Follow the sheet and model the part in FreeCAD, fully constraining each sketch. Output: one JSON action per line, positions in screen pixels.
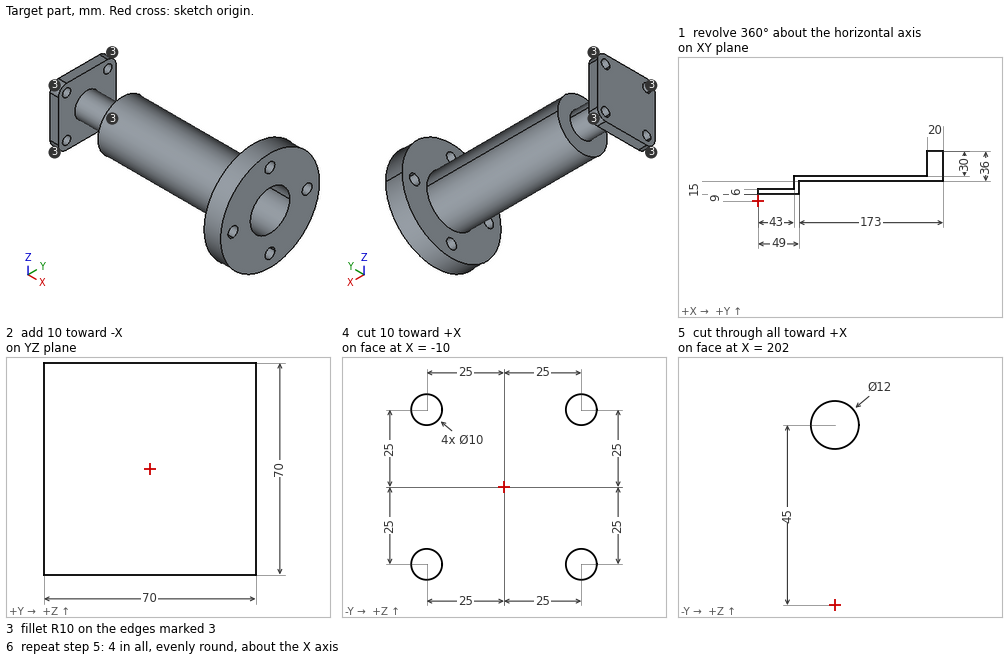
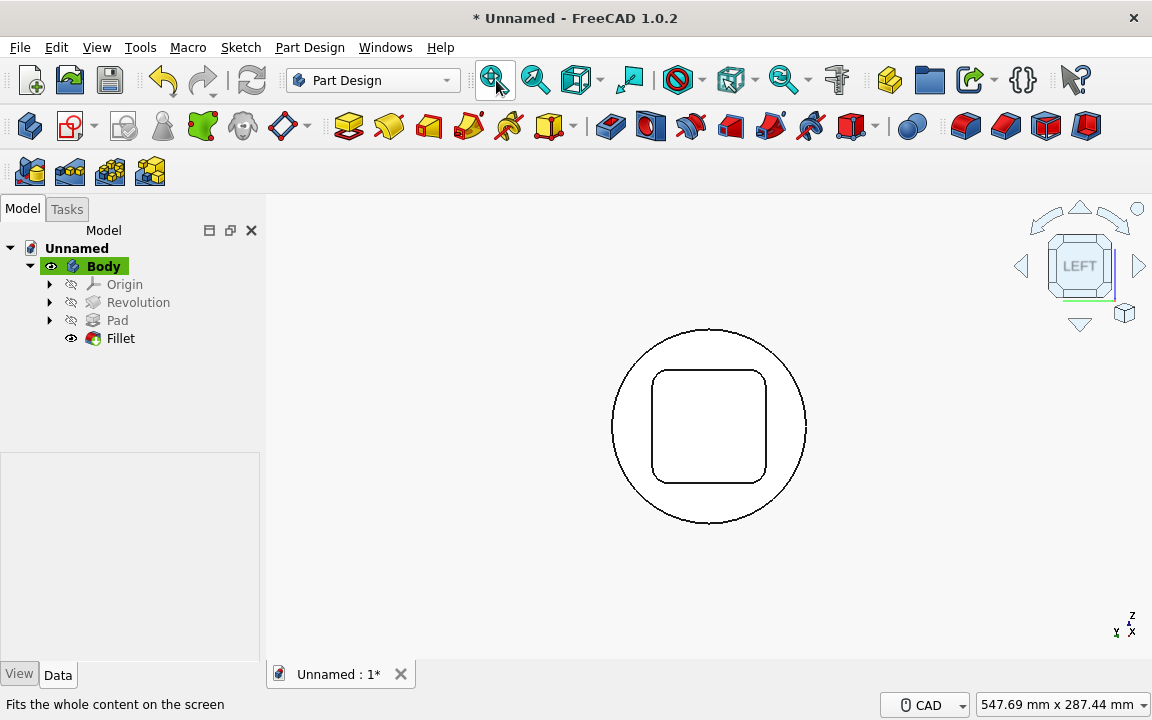
{"action": "left_click", "coordinate": [709, 425]}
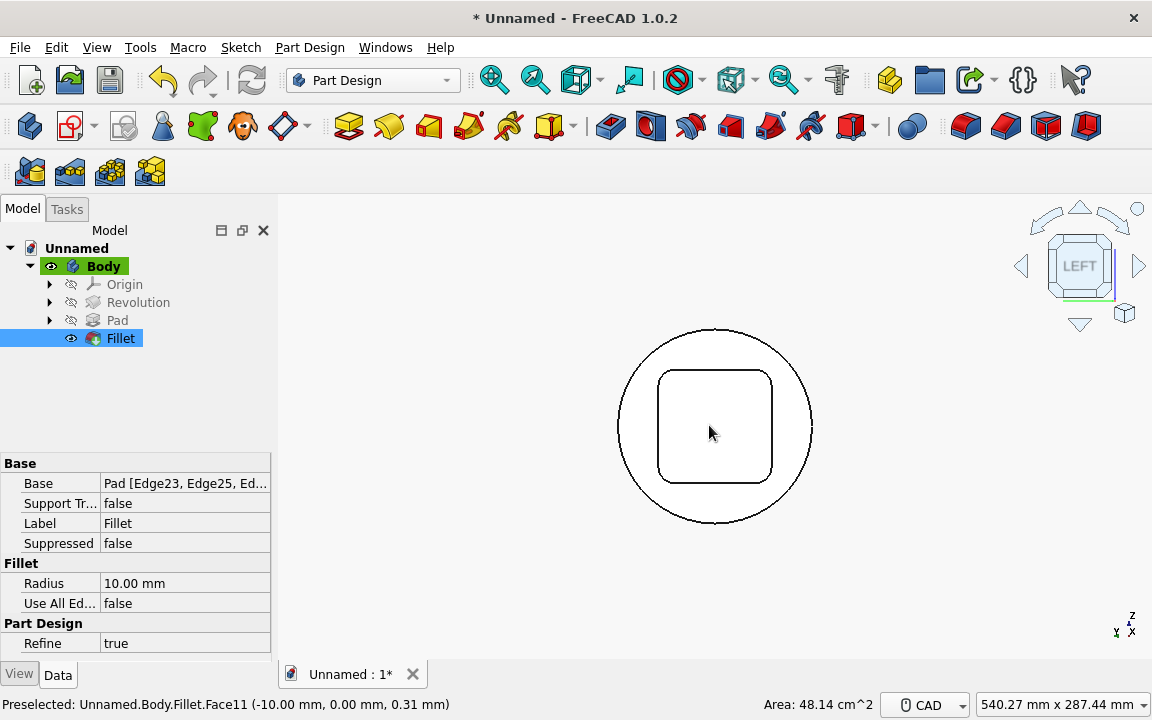
{"action": "left_click", "coordinate": [70, 126]}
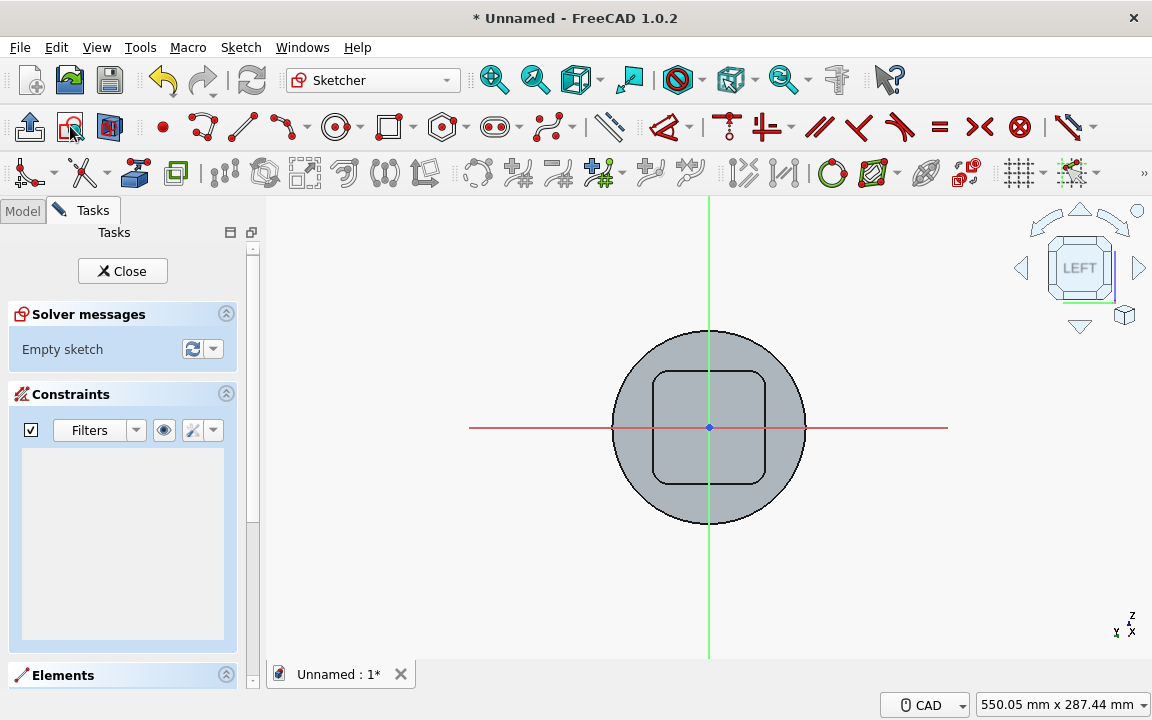
{"action": "scroll", "coordinate": [749, 428], "scroll_direction": "up", "scroll_amount": 5}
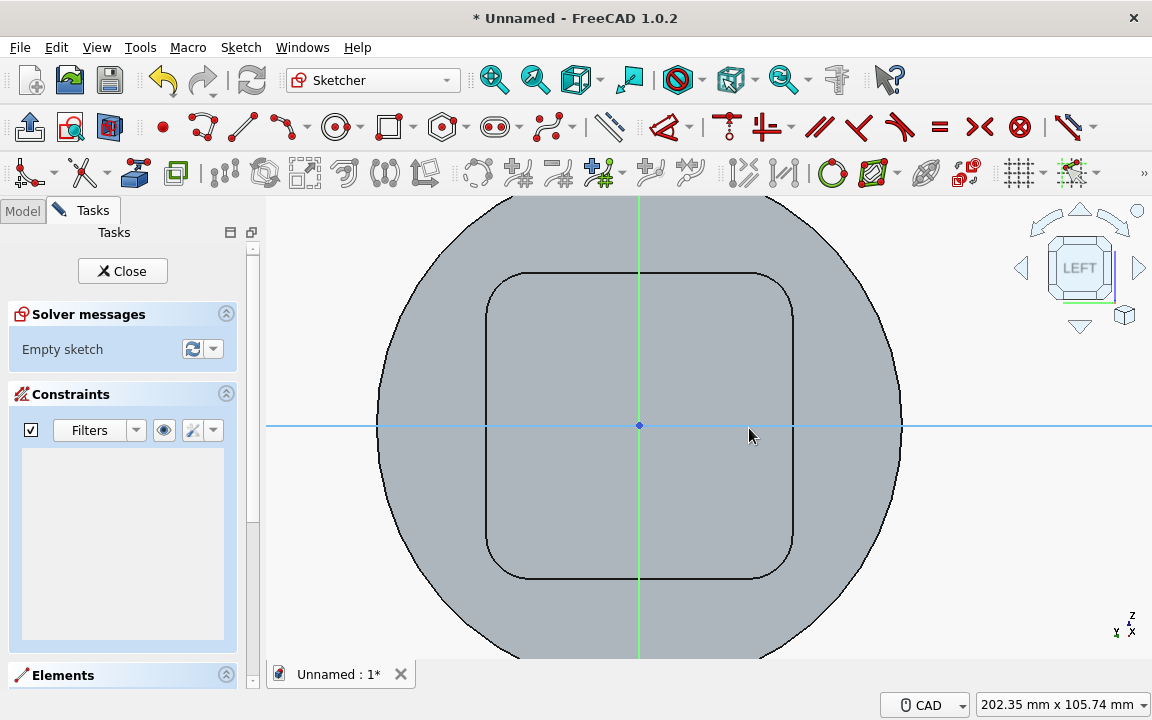
{"action": "key", "text": "g c"}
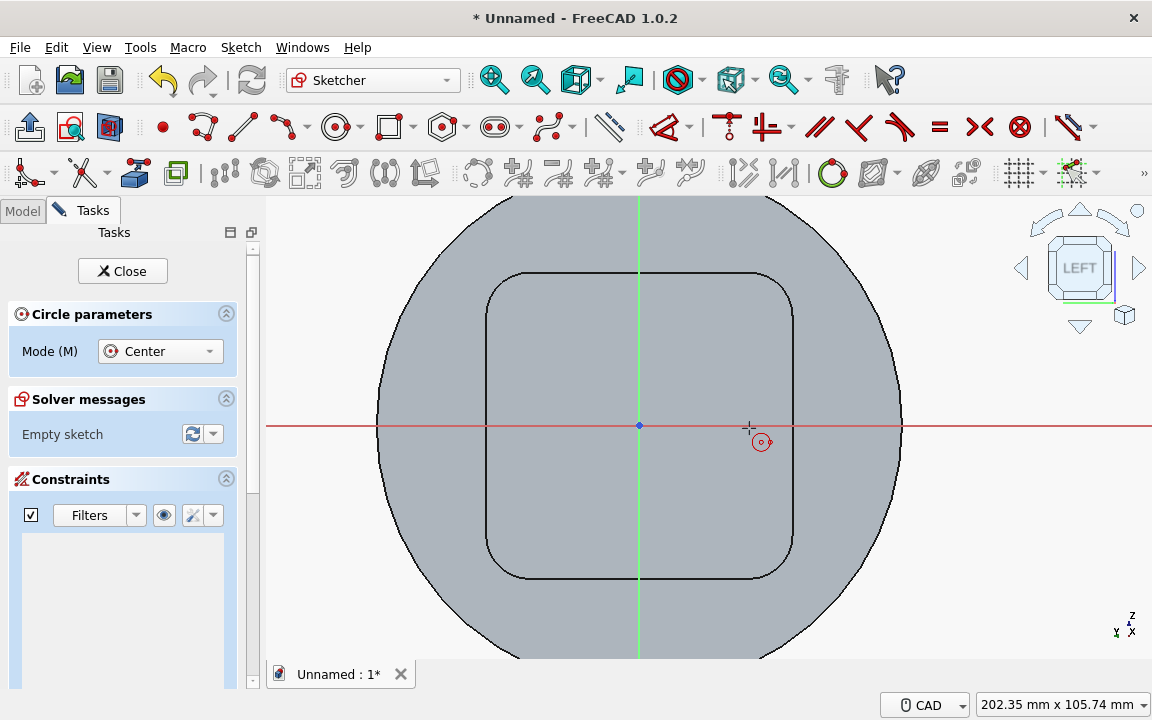
{"action": "left_click", "coordinate": [530, 316]}
{"action": "mouse_move", "coordinate": [545, 301]}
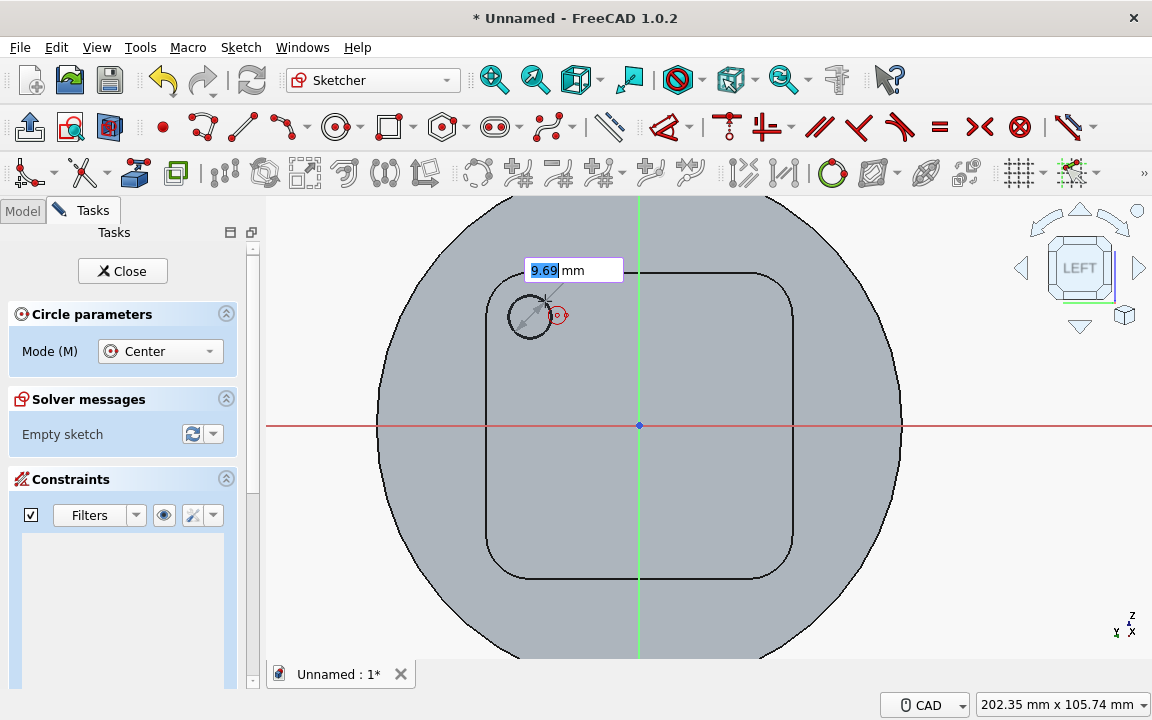
{"action": "type", "text": "10"}
{"action": "key", "text": "Return"}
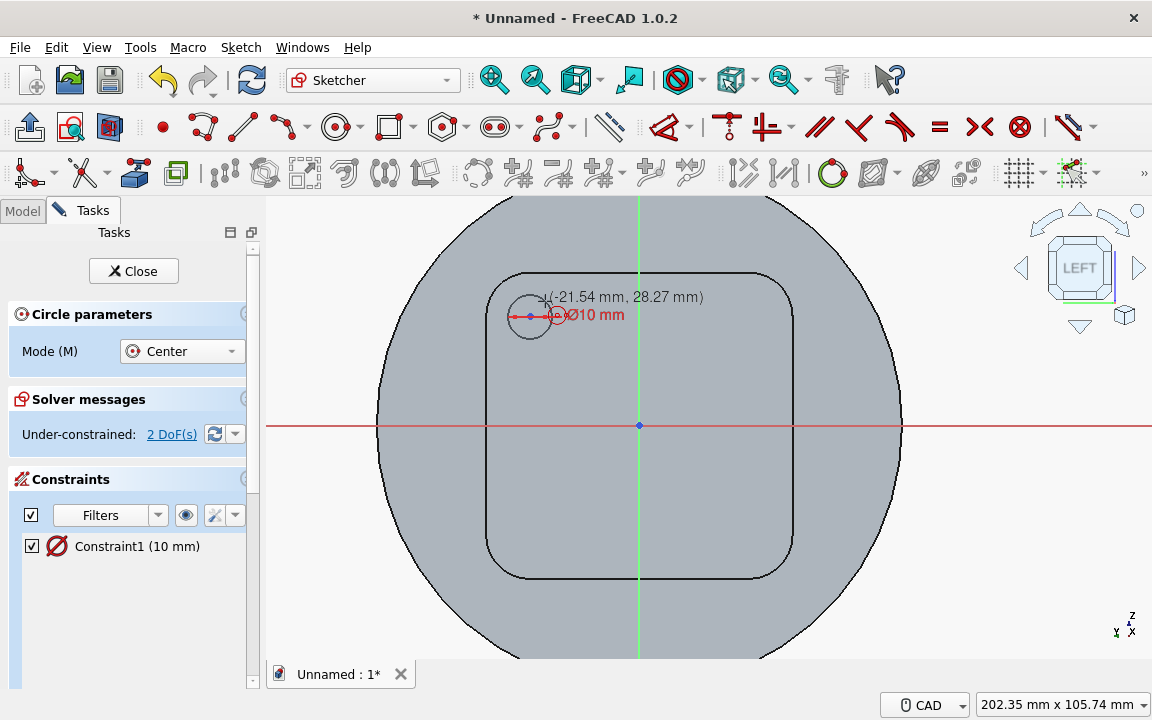
{"action": "left_click", "coordinate": [530, 535]}
{"action": "mouse_move", "coordinate": [545, 520]}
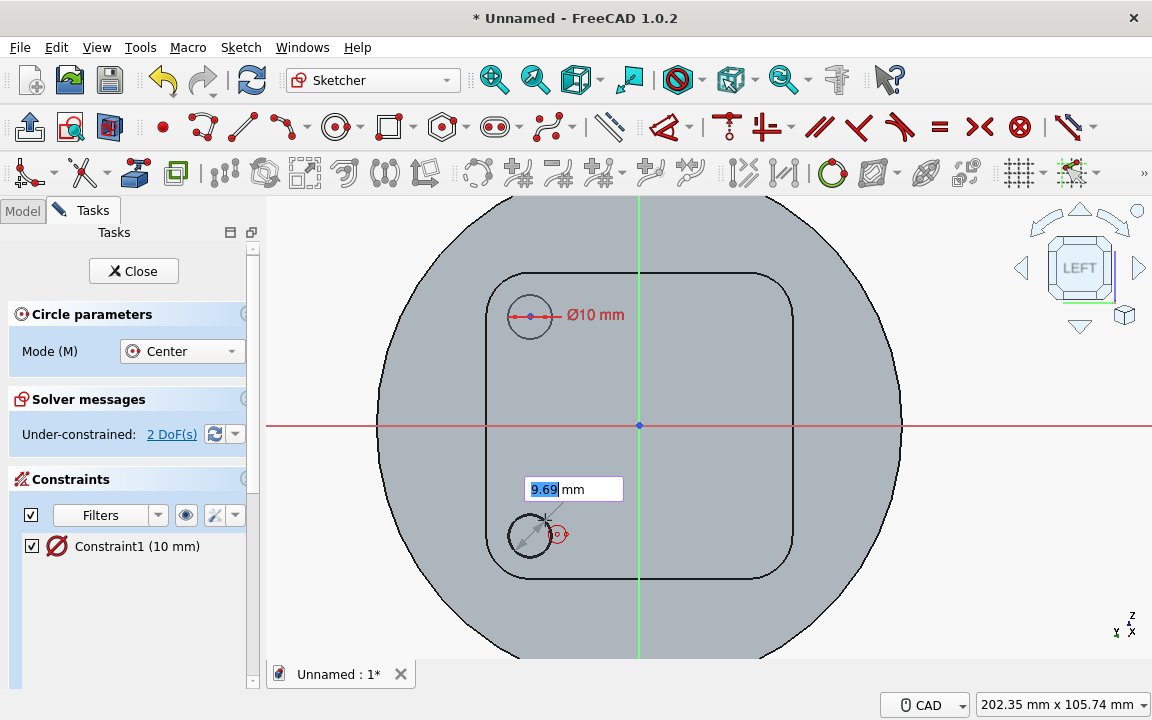
{"action": "type", "text": "10"}
{"action": "key", "text": "Return"}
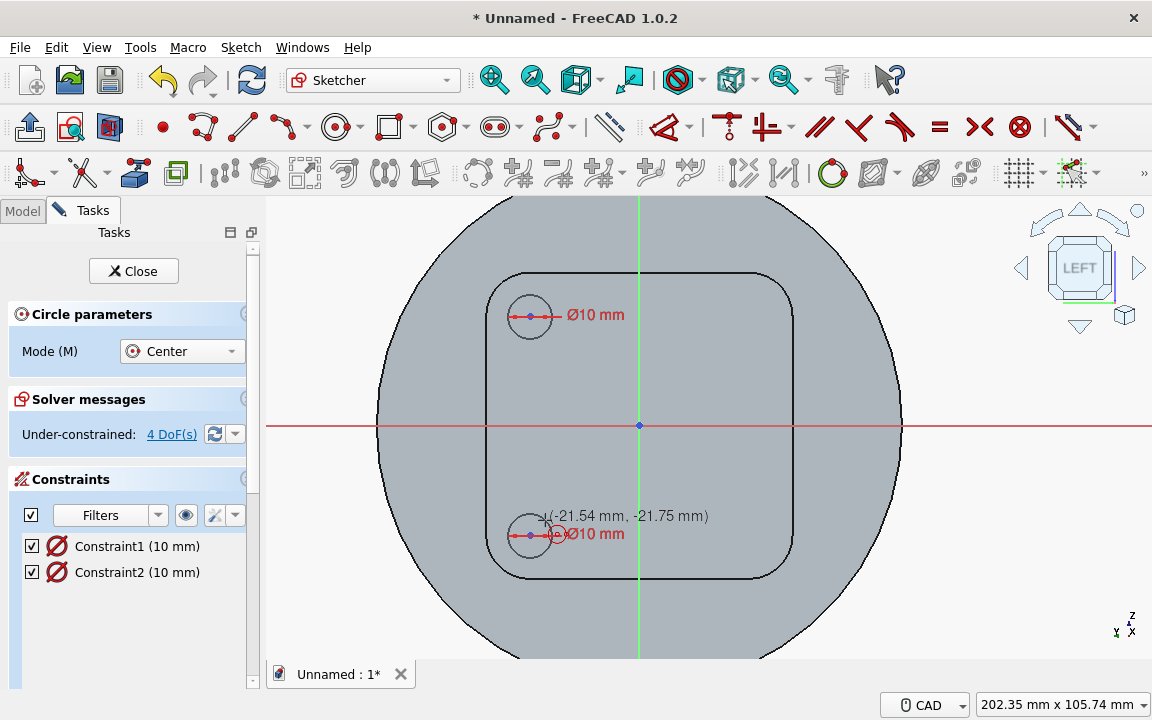
{"action": "left_click", "coordinate": [749, 535]}
{"action": "mouse_move", "coordinate": [764, 520]}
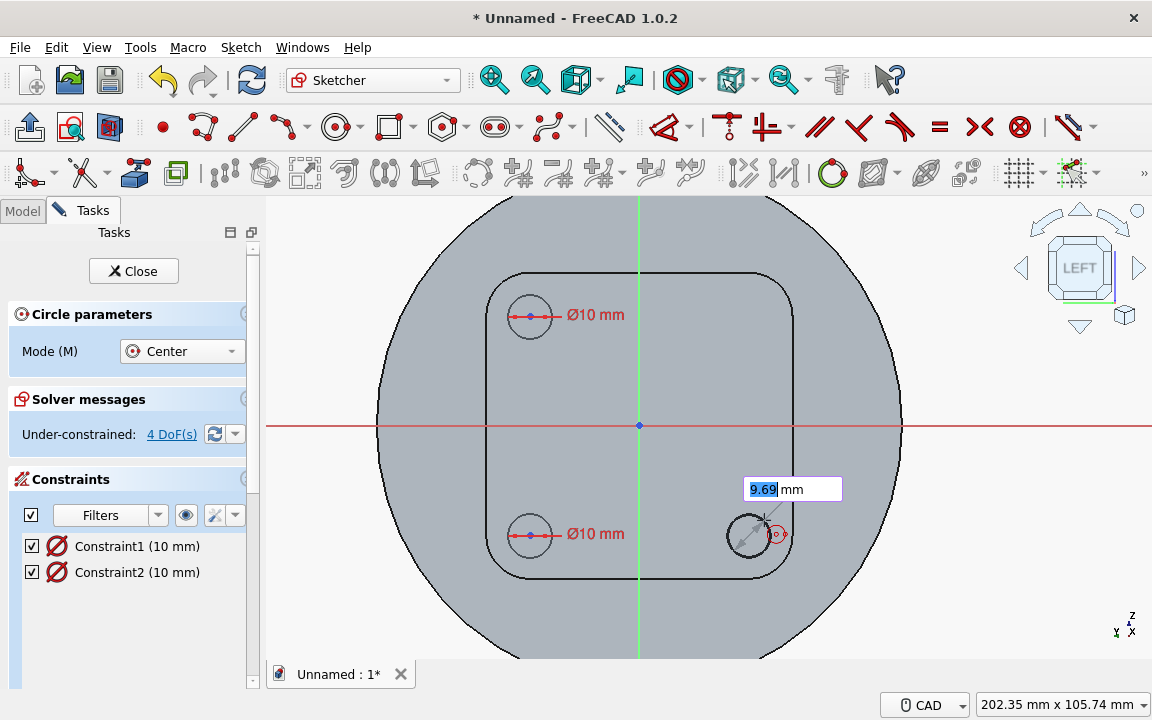
{"action": "type", "text": "10"}
{"action": "key", "text": "Return"}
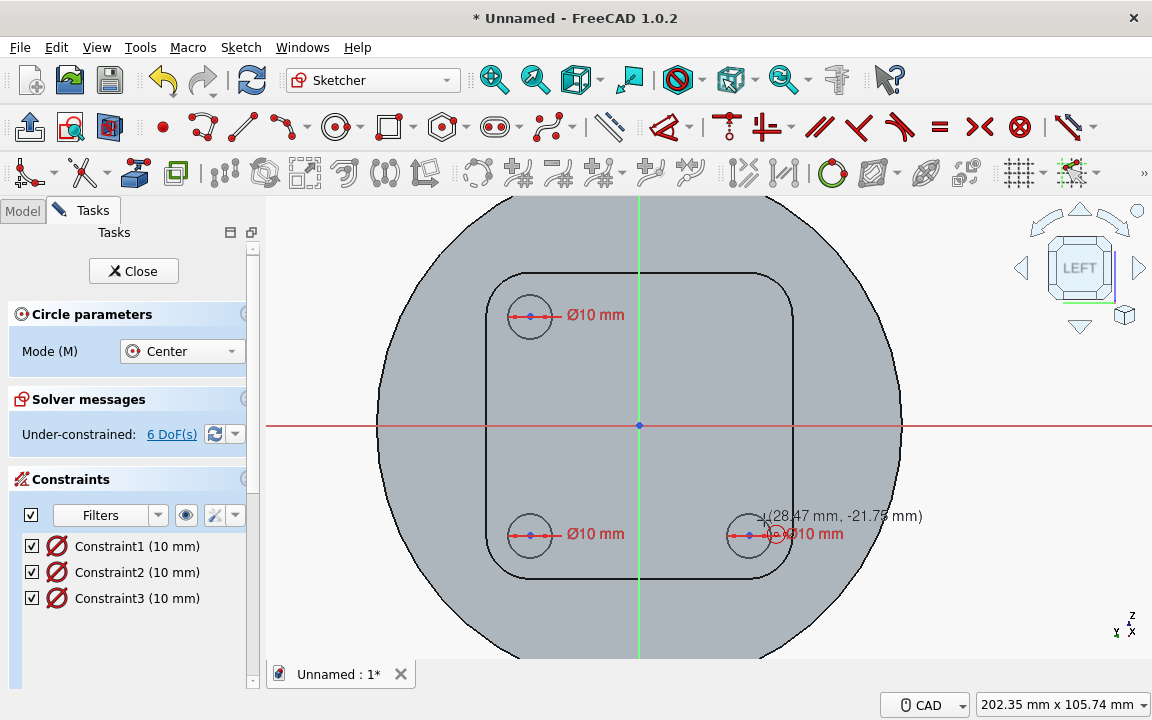
{"action": "left_click", "coordinate": [749, 316]}
{"action": "mouse_move", "coordinate": [764, 301]}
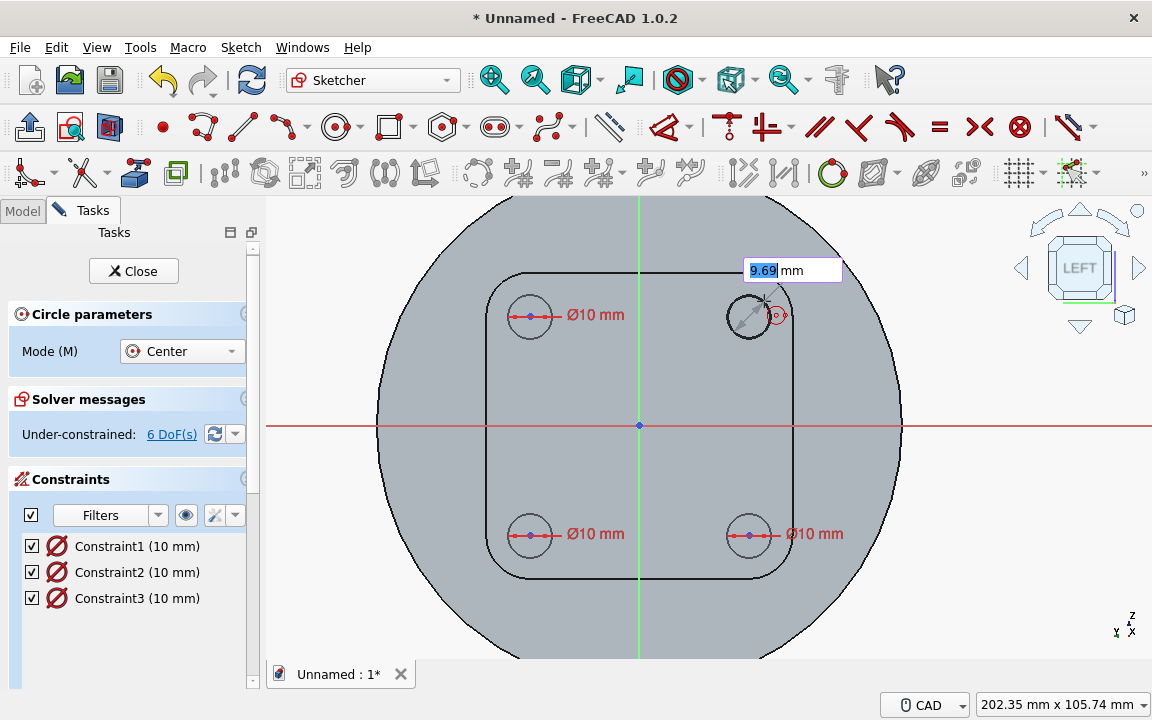
{"action": "type", "text": "10"}
{"action": "key", "text": "Return"}
{"action": "key", "text": "Escape"}